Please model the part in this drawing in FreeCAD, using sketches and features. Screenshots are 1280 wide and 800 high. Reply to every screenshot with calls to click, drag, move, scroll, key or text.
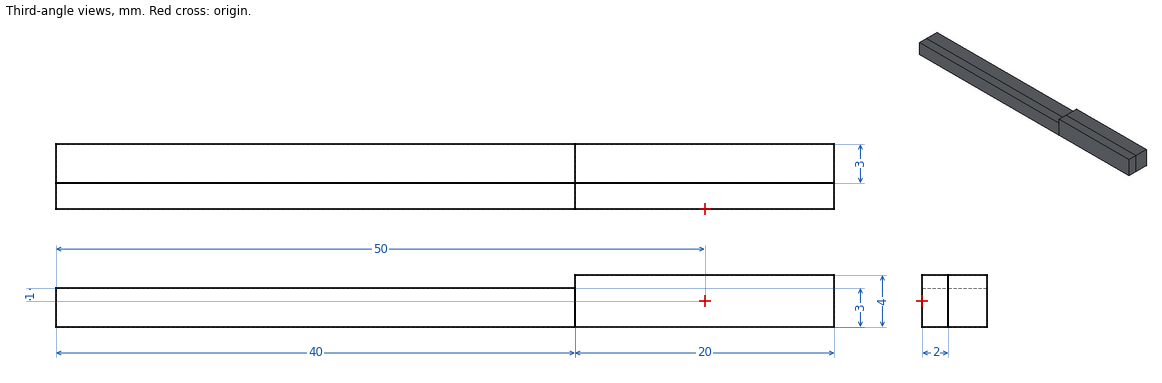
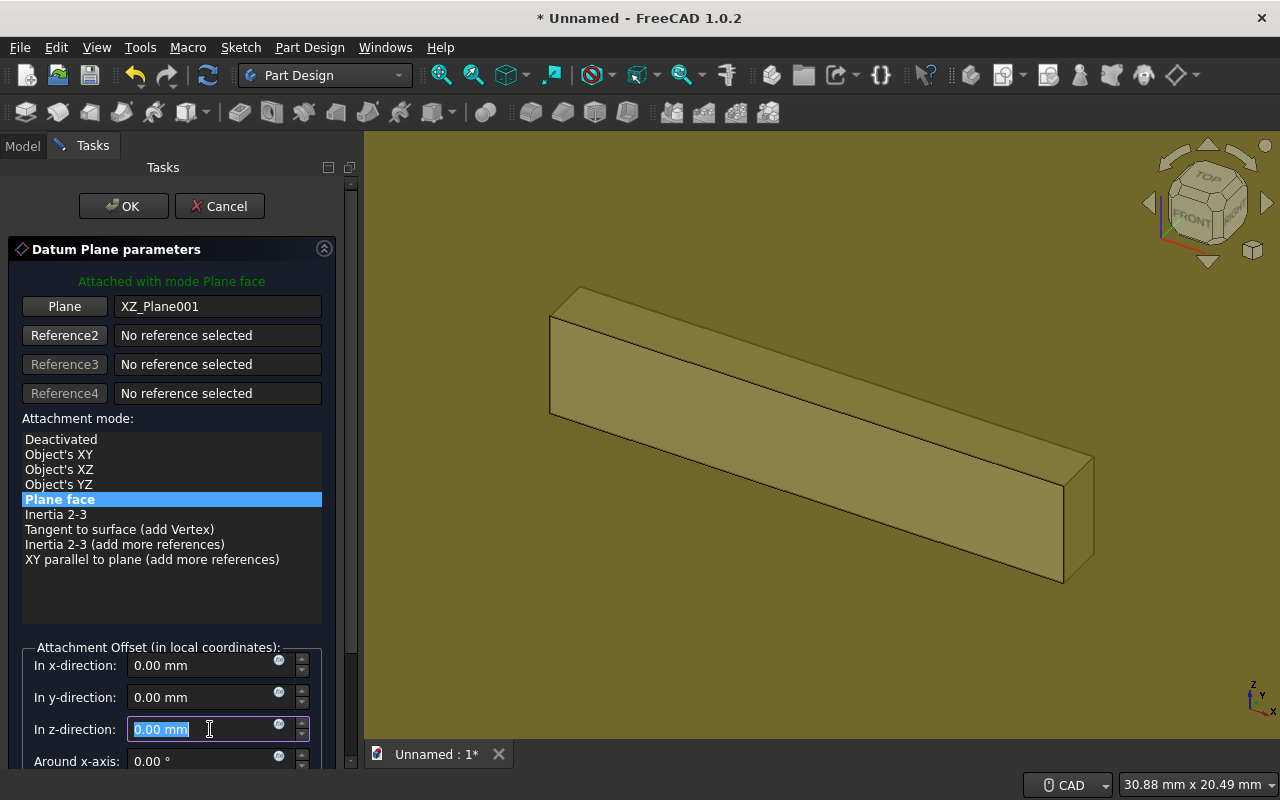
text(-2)
key(Tab)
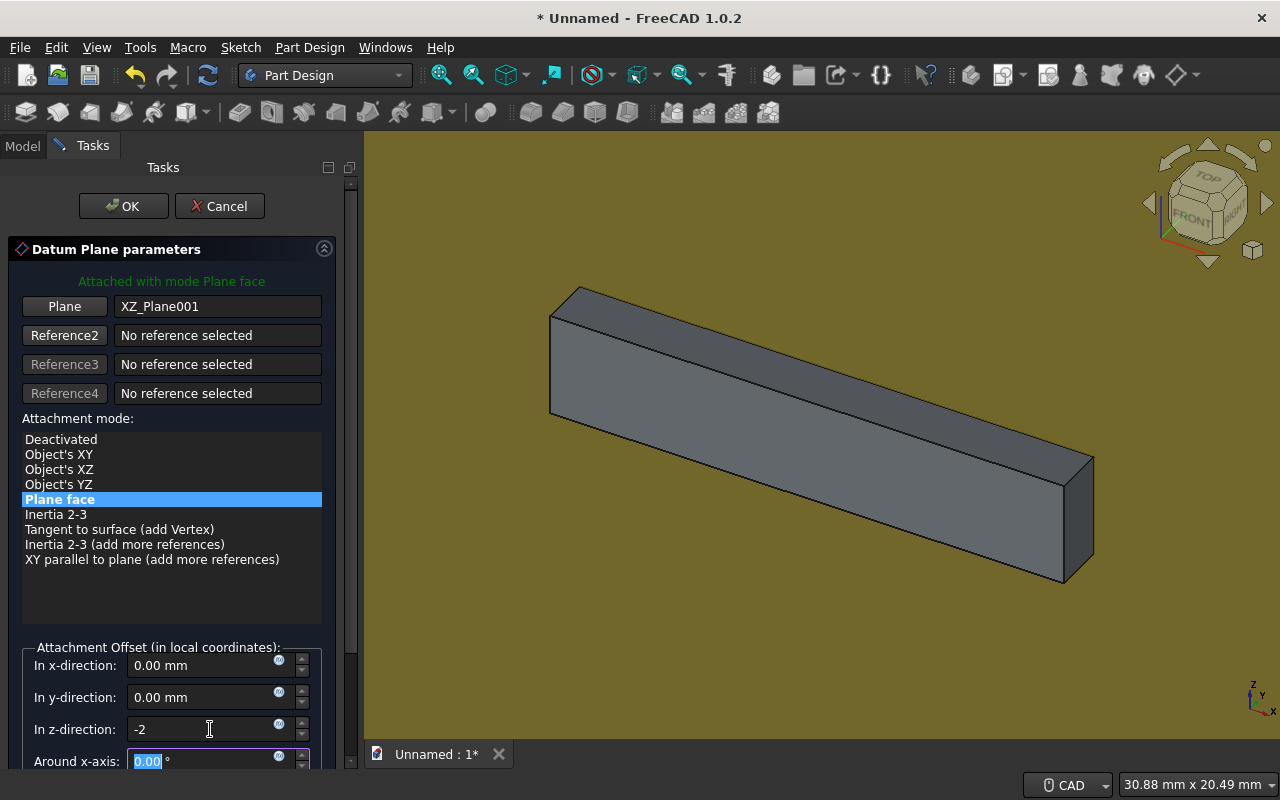
click(124, 206)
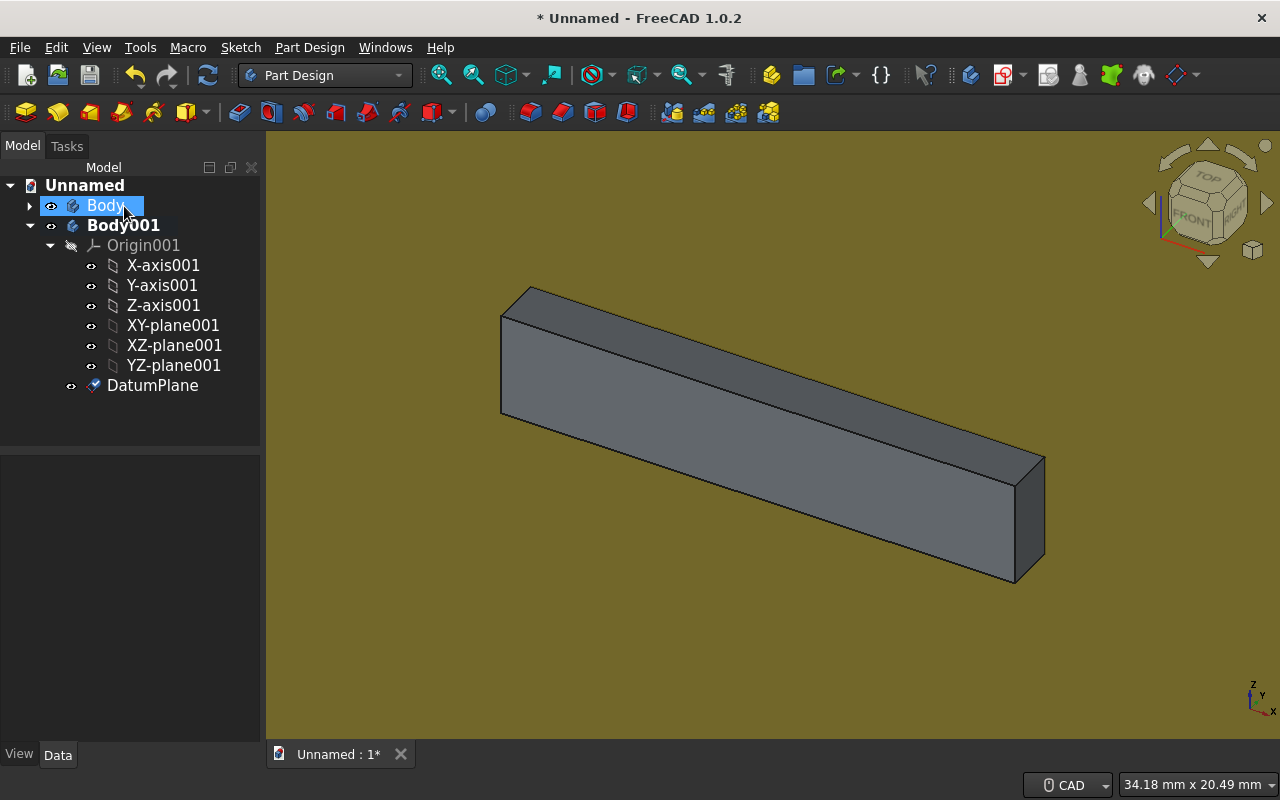
click(116, 386)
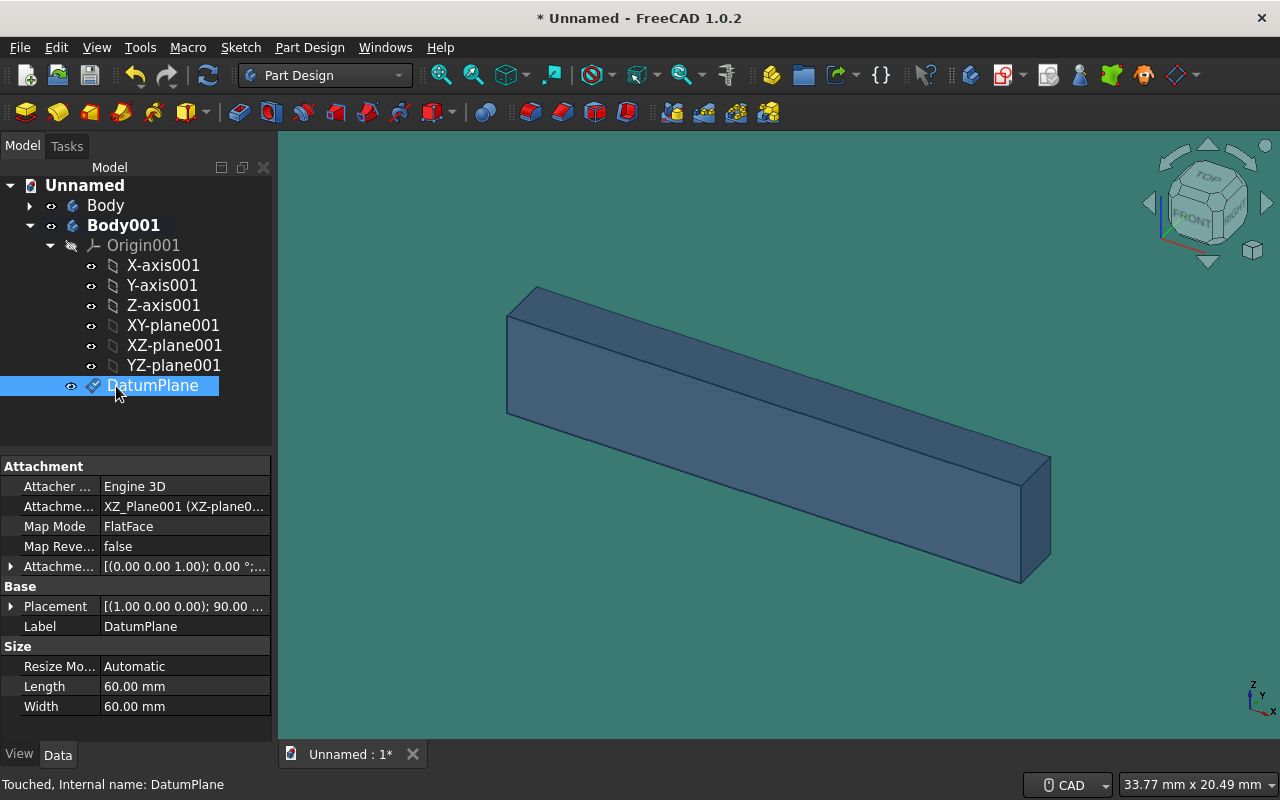
click(1004, 76)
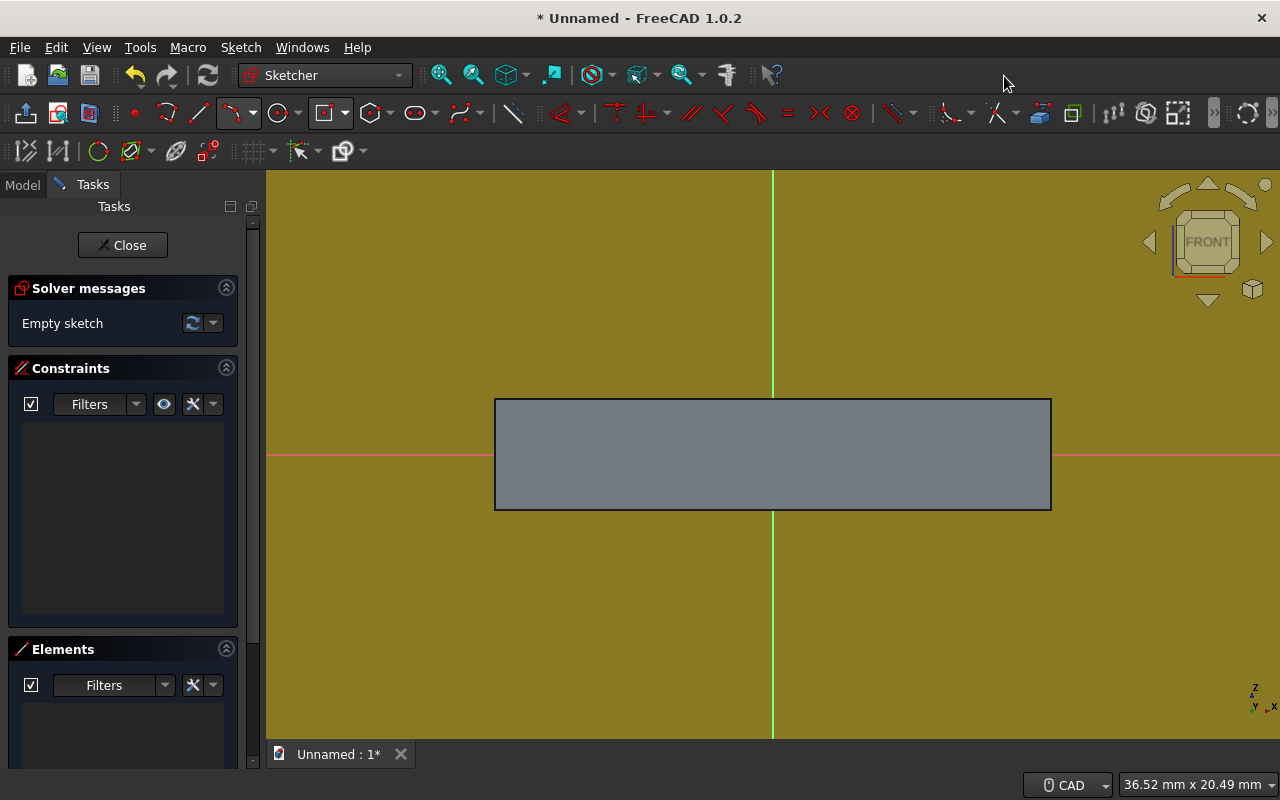
key(g)
key(v)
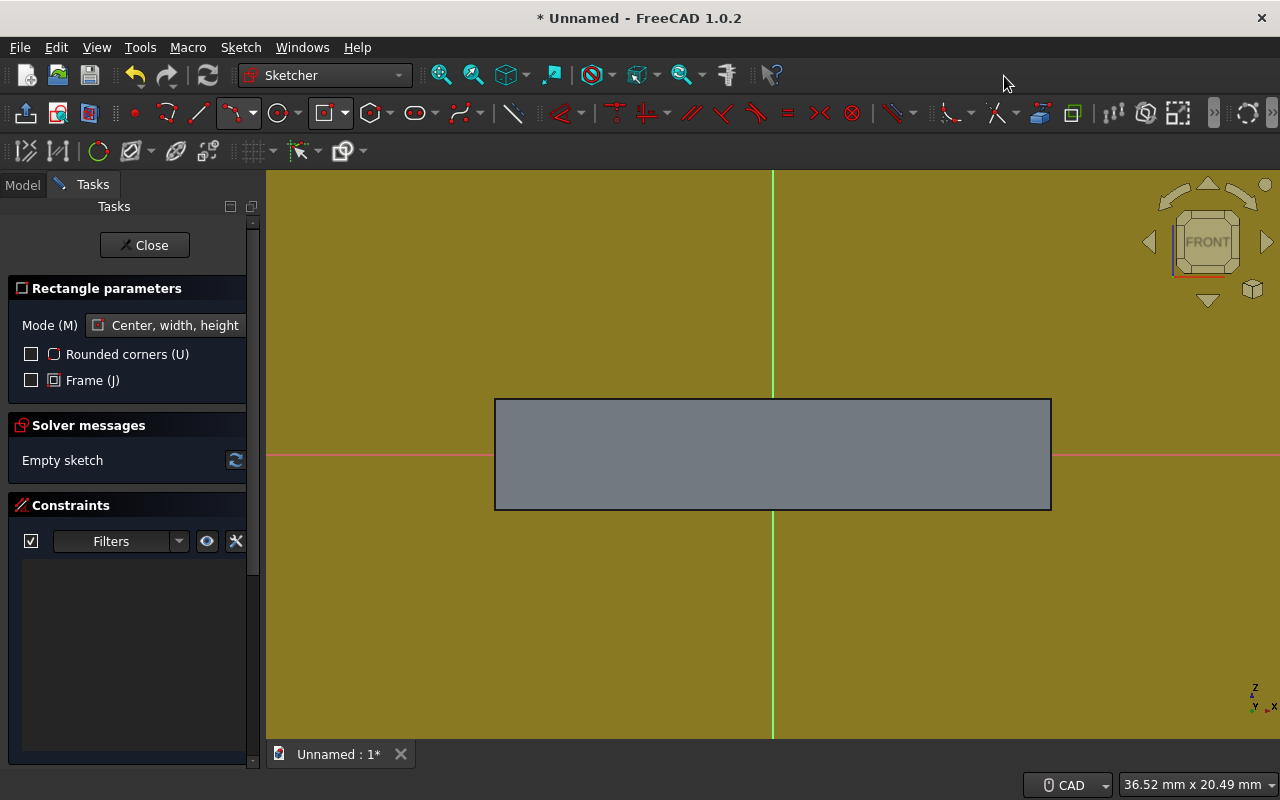
click(773, 454)
move(1051, 399)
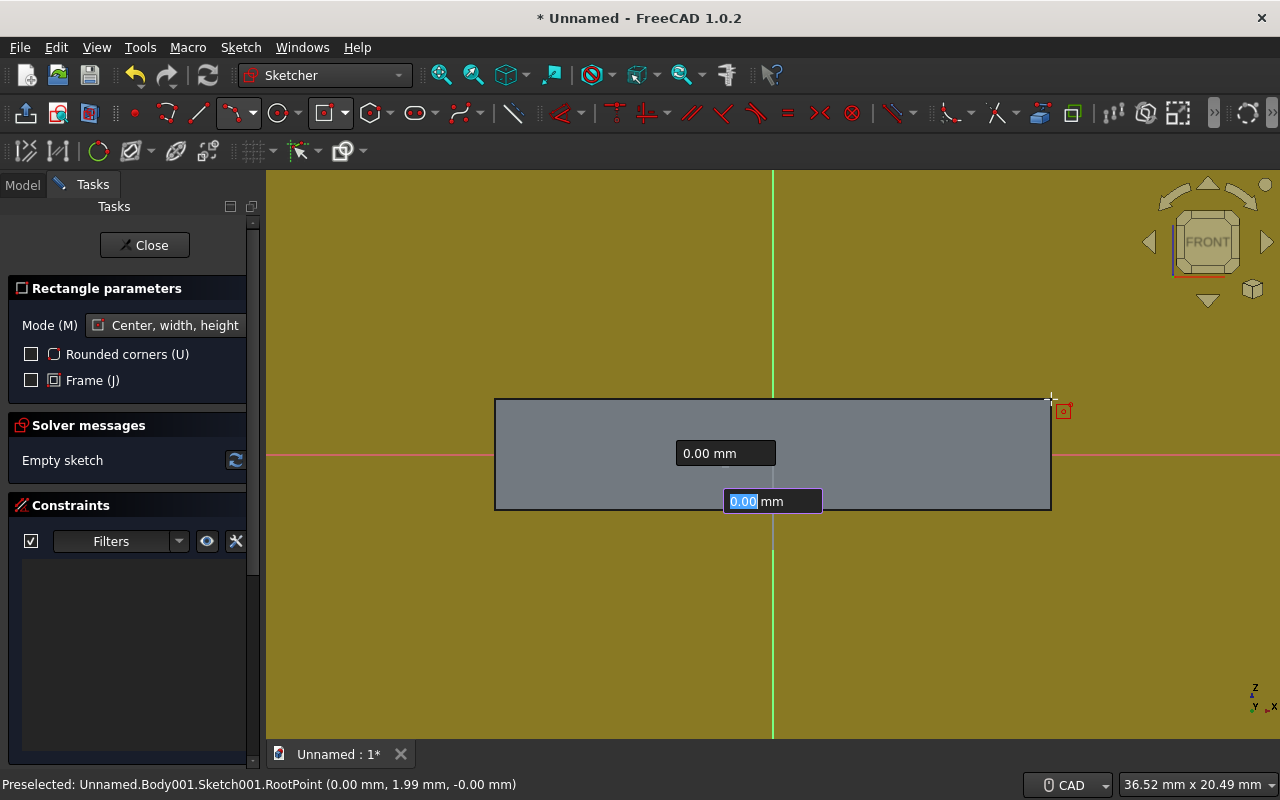
text(20)
key(Tab)
text(4)
key(Return)
key(Escape)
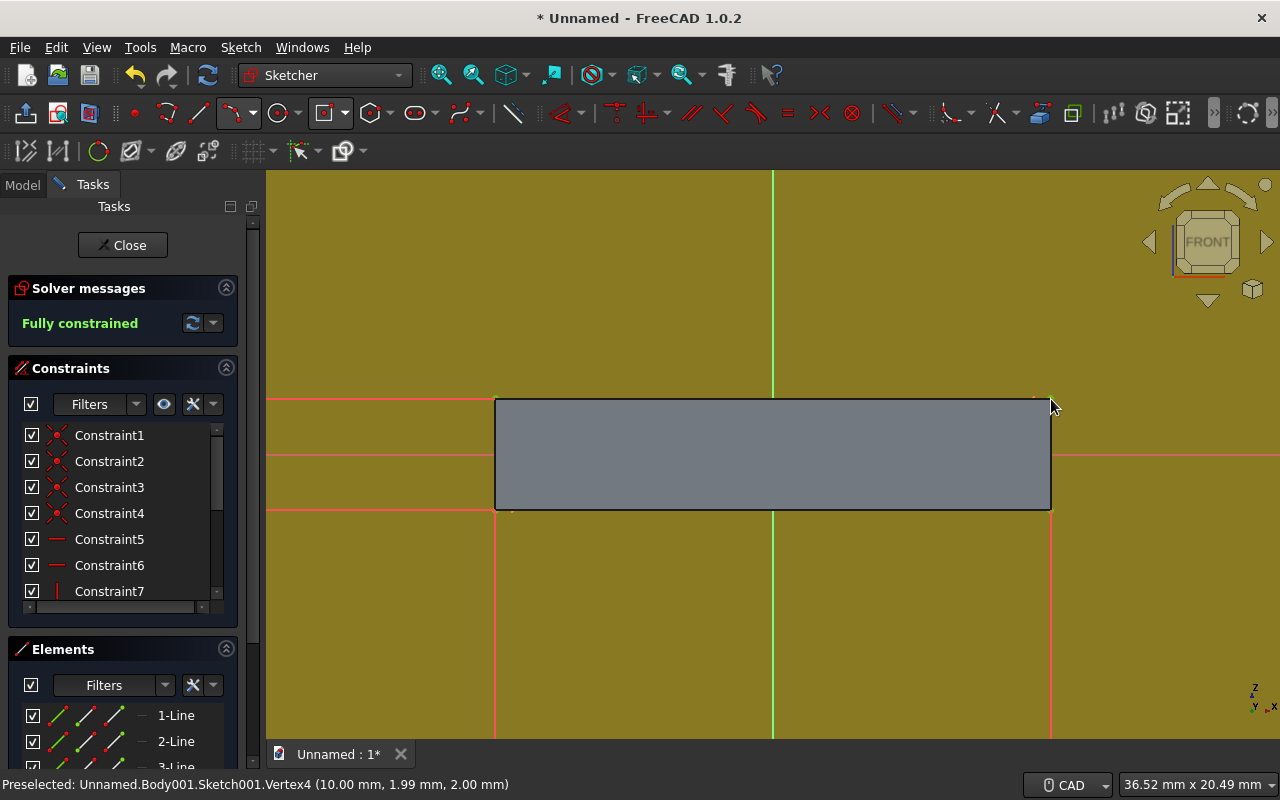
click(123, 245)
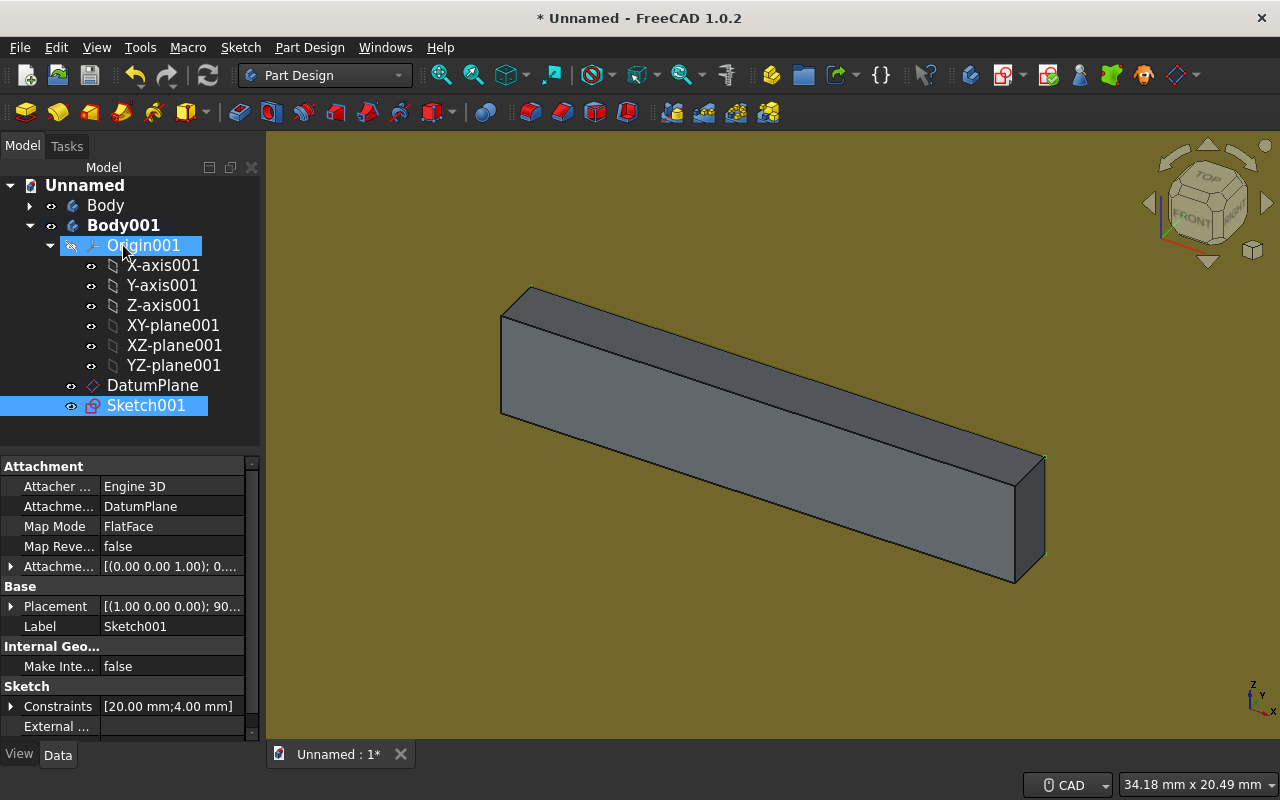
click(26, 112)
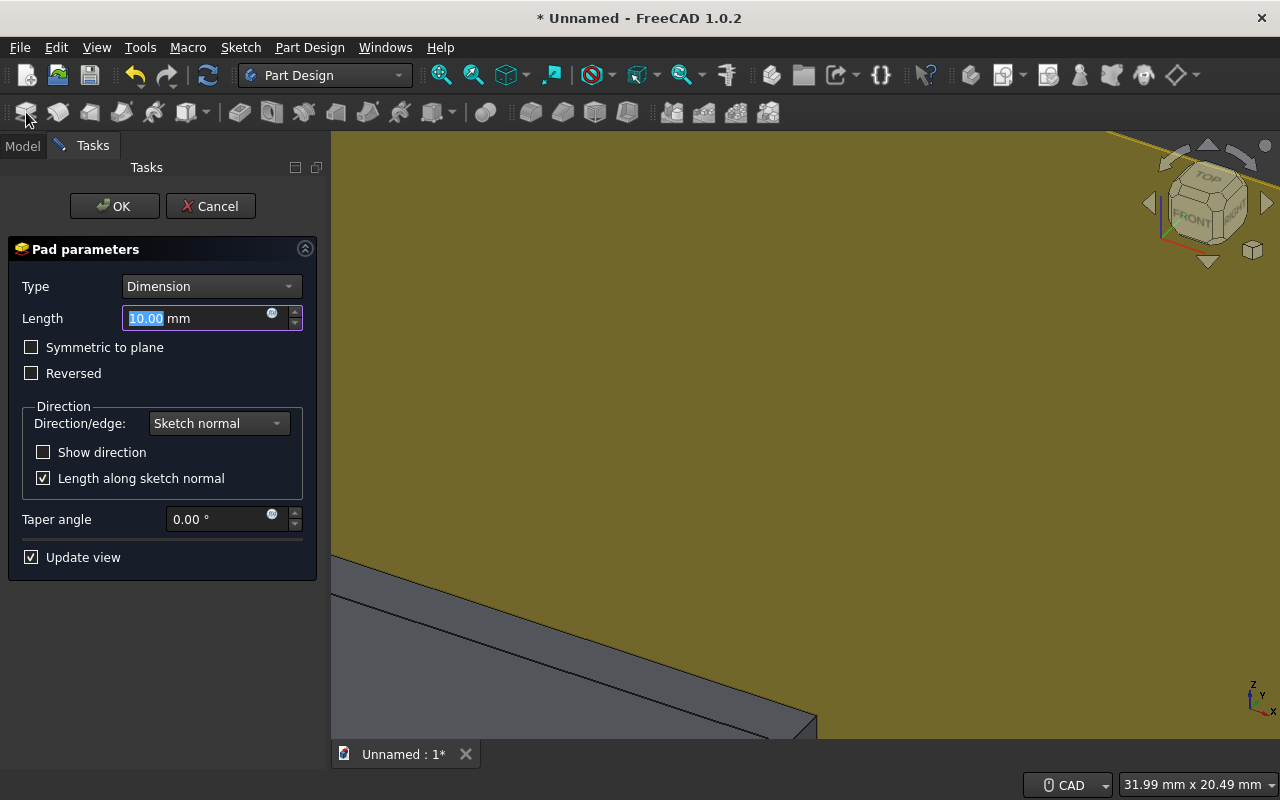
text(3)
key(Tab)